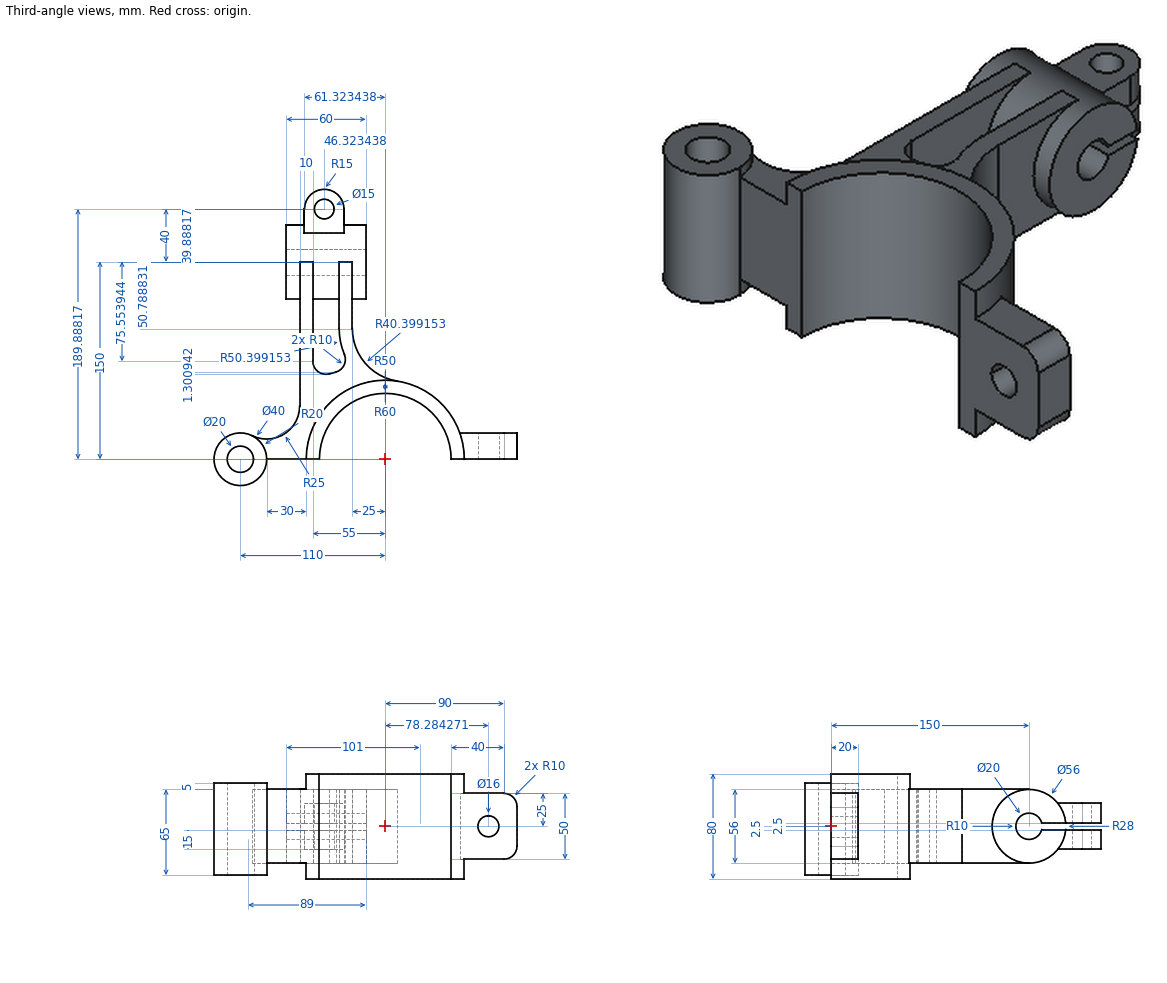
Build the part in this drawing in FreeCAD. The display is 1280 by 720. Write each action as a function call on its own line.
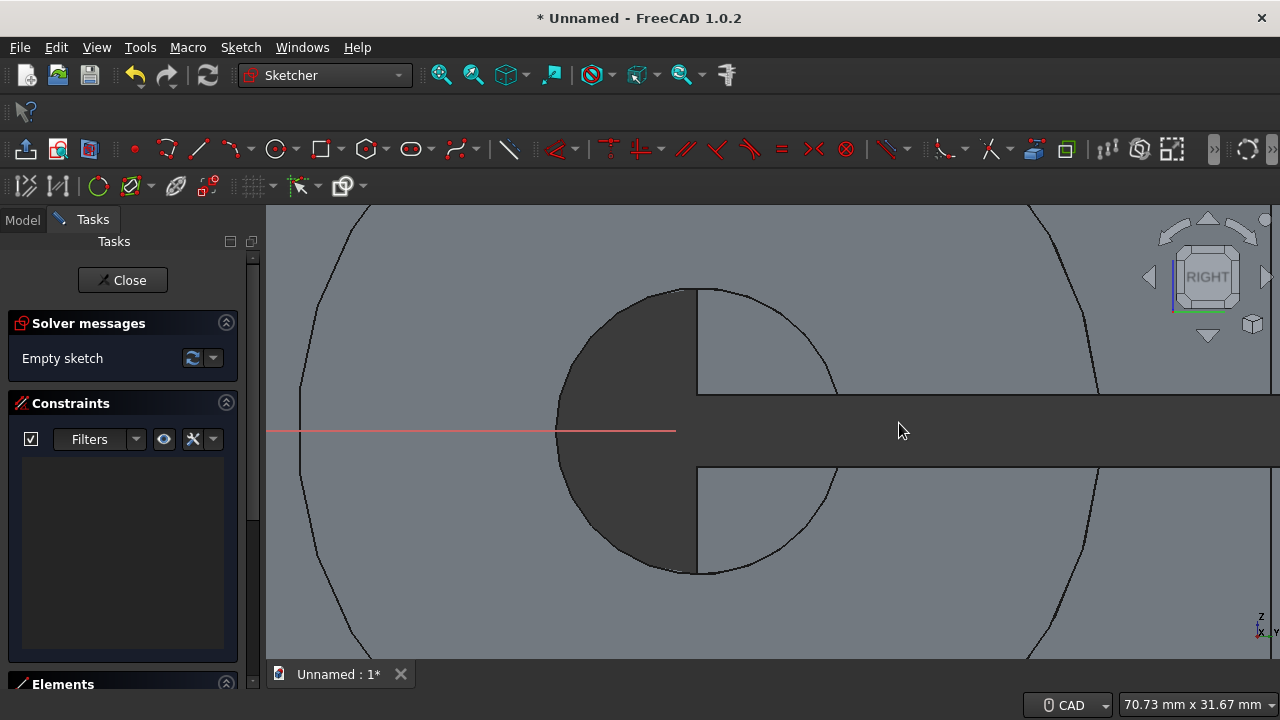
key(g)
key(c)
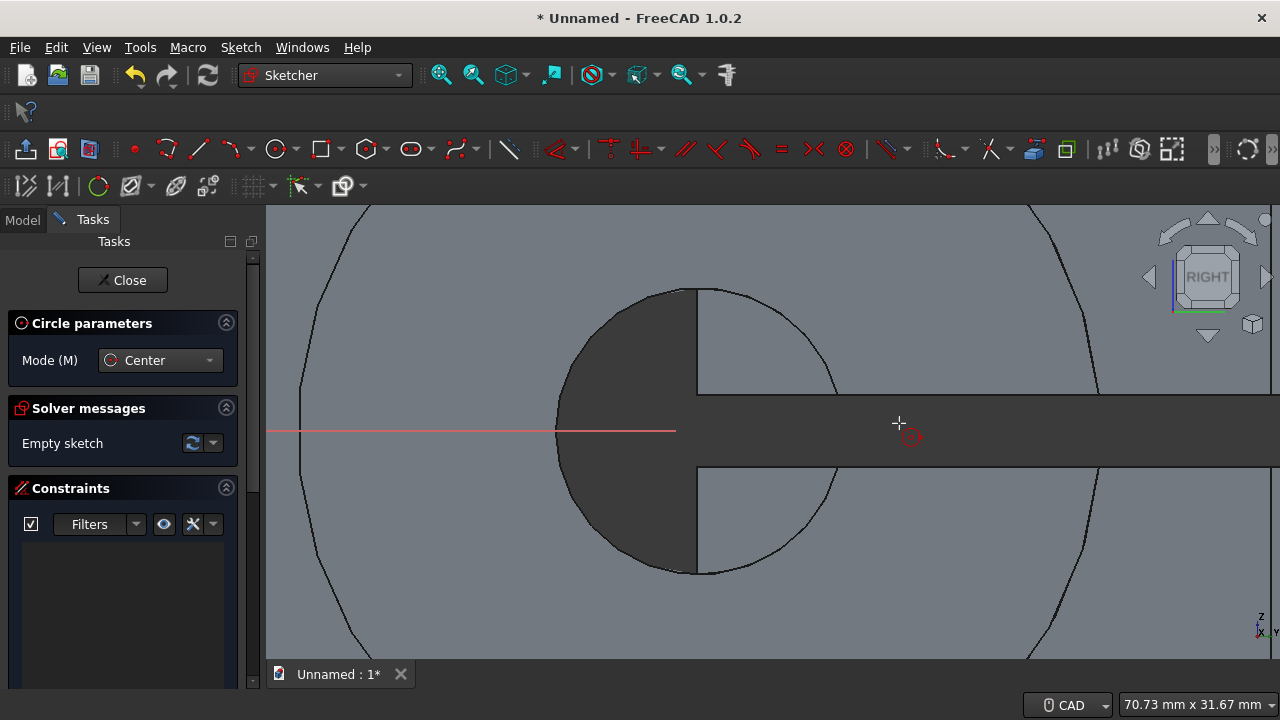
click(699, 431)
move(800, 330)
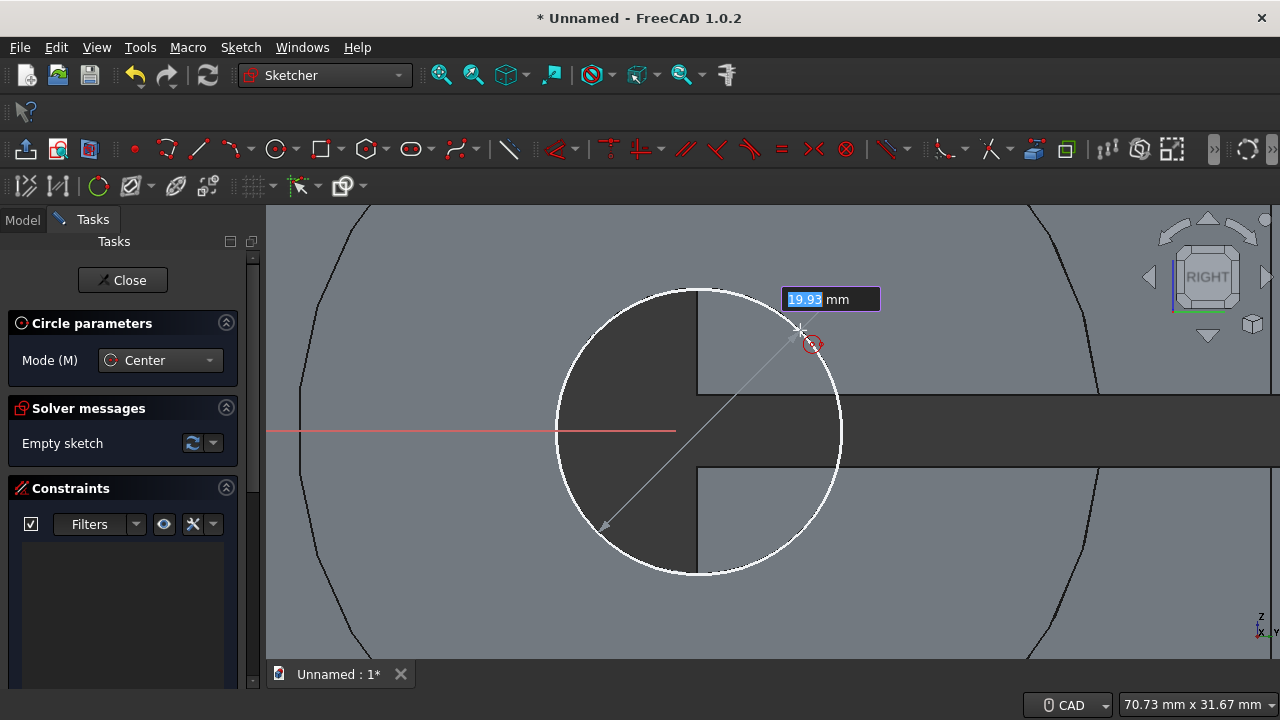
text(20)
key(Return)
key(Escape)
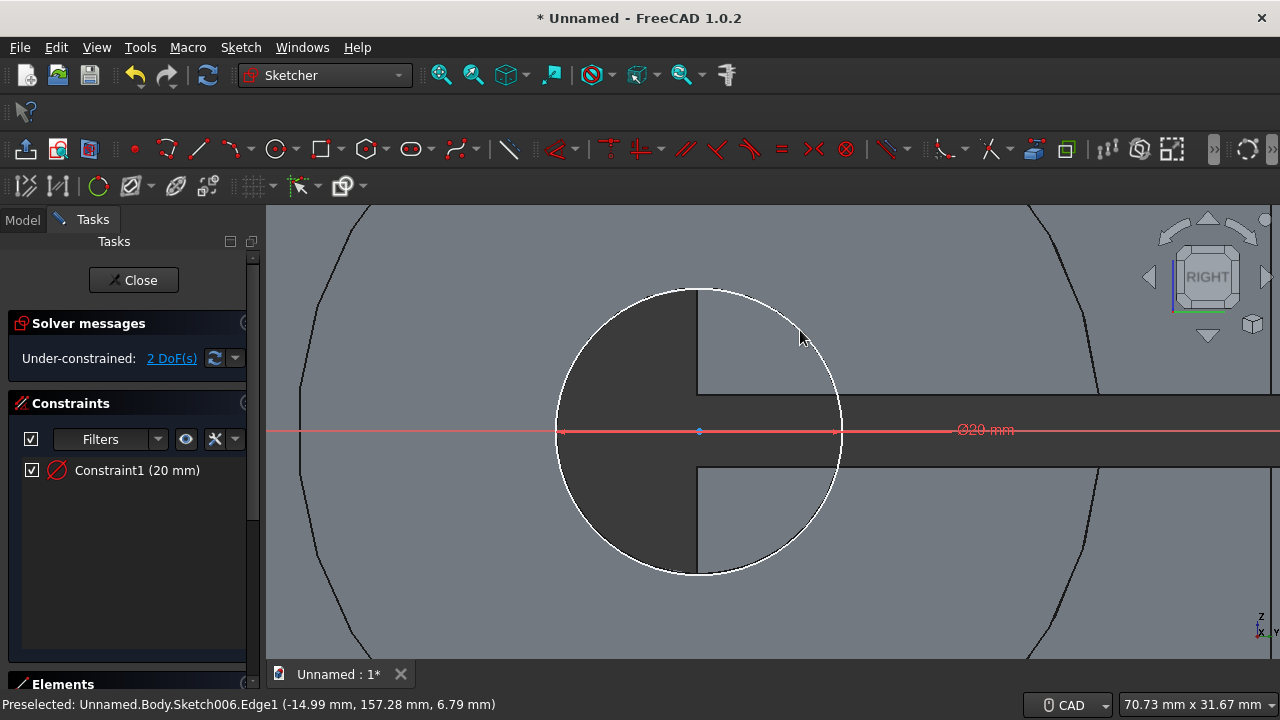
click(699, 432)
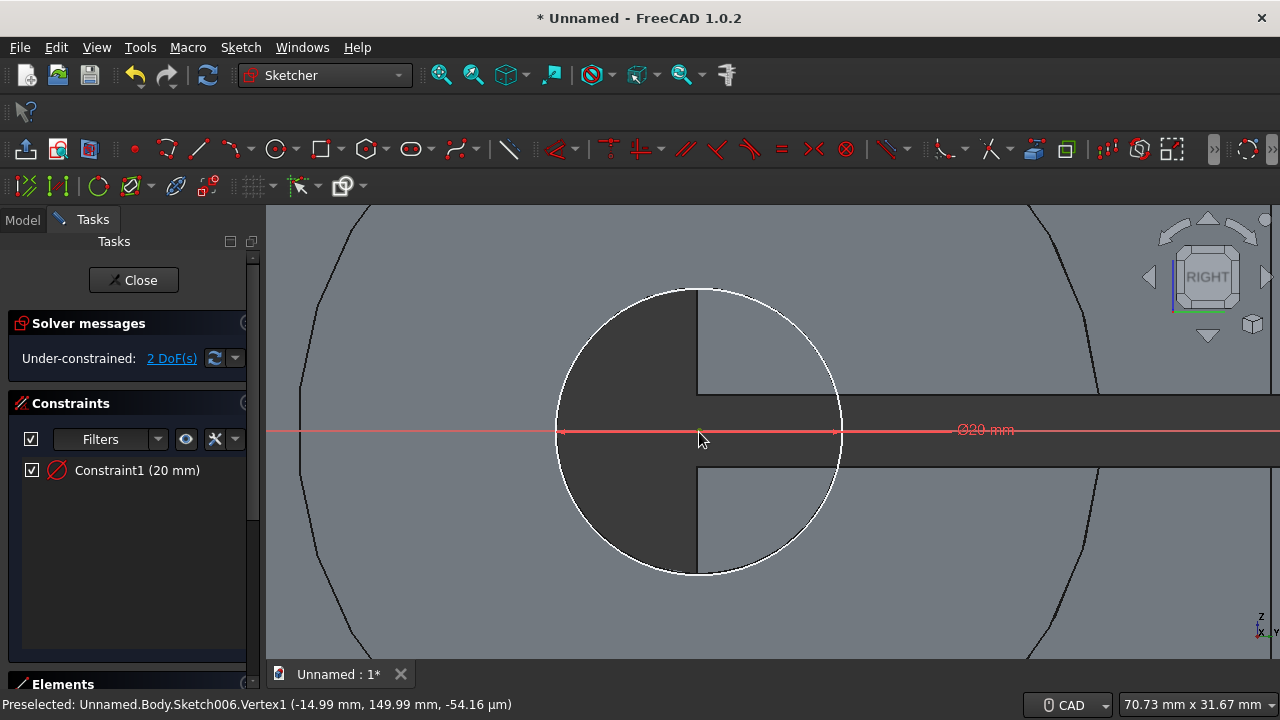
click(353, 431)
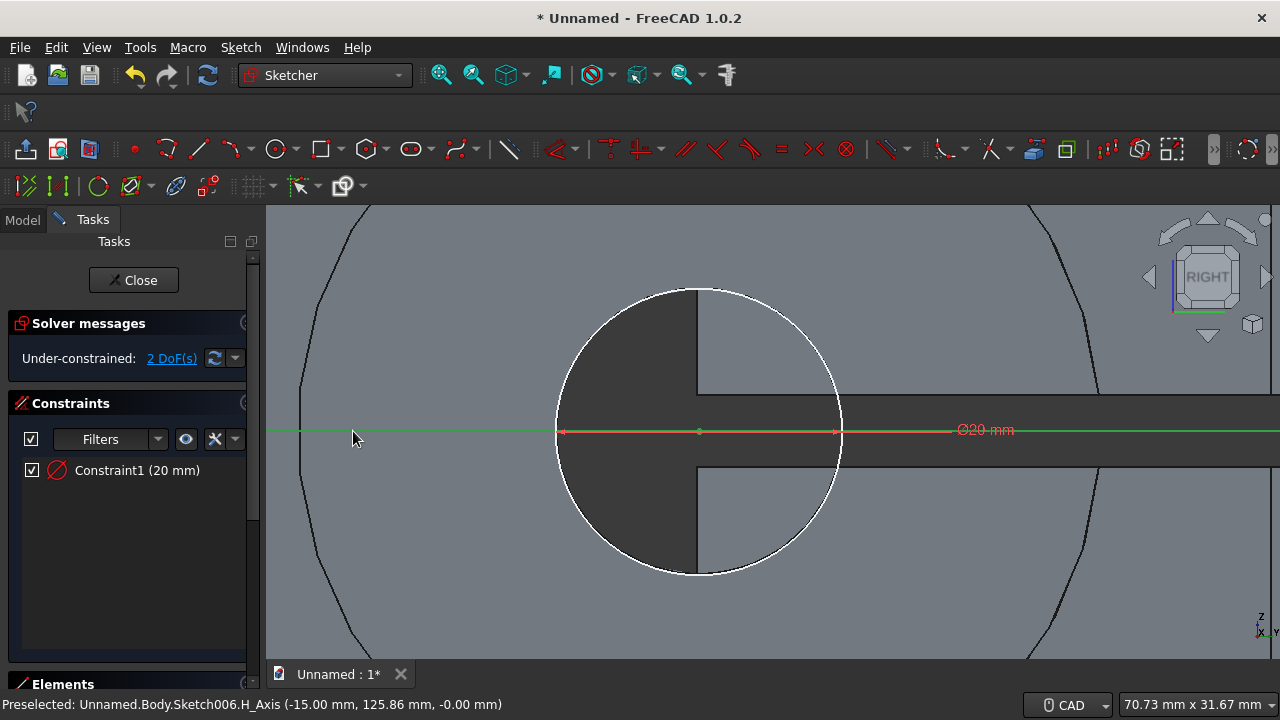
key(c)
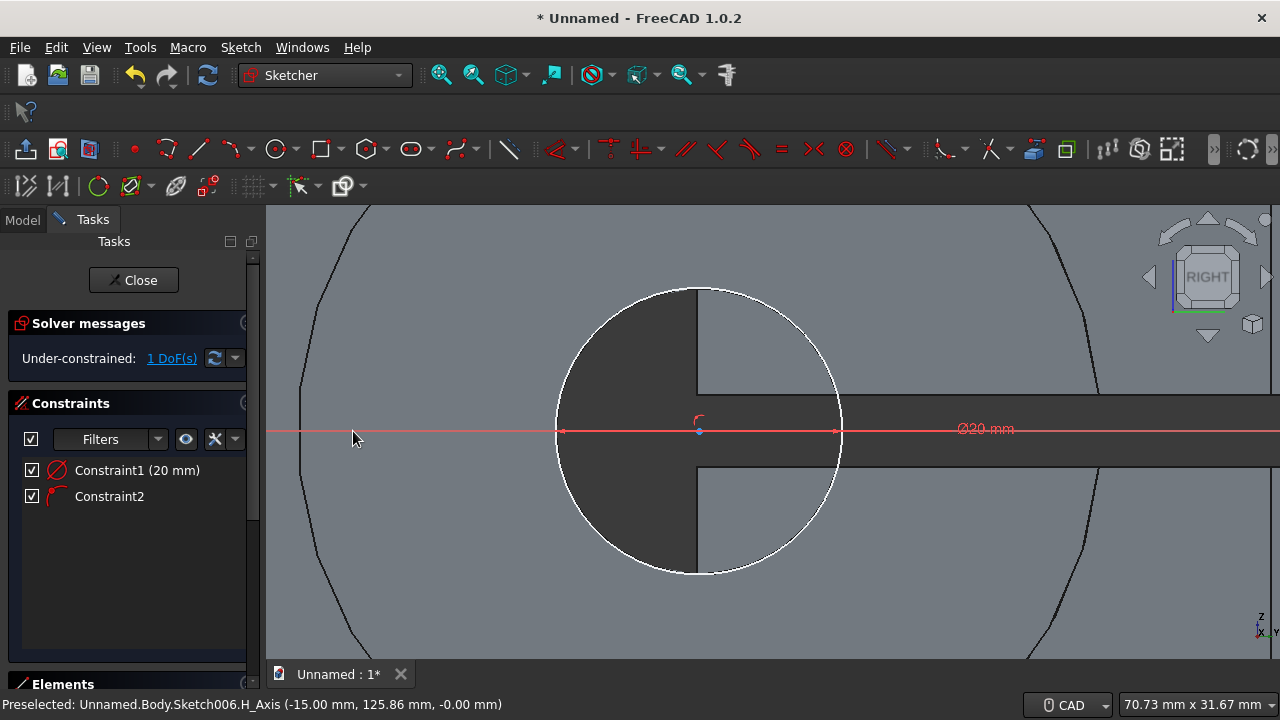
key(d)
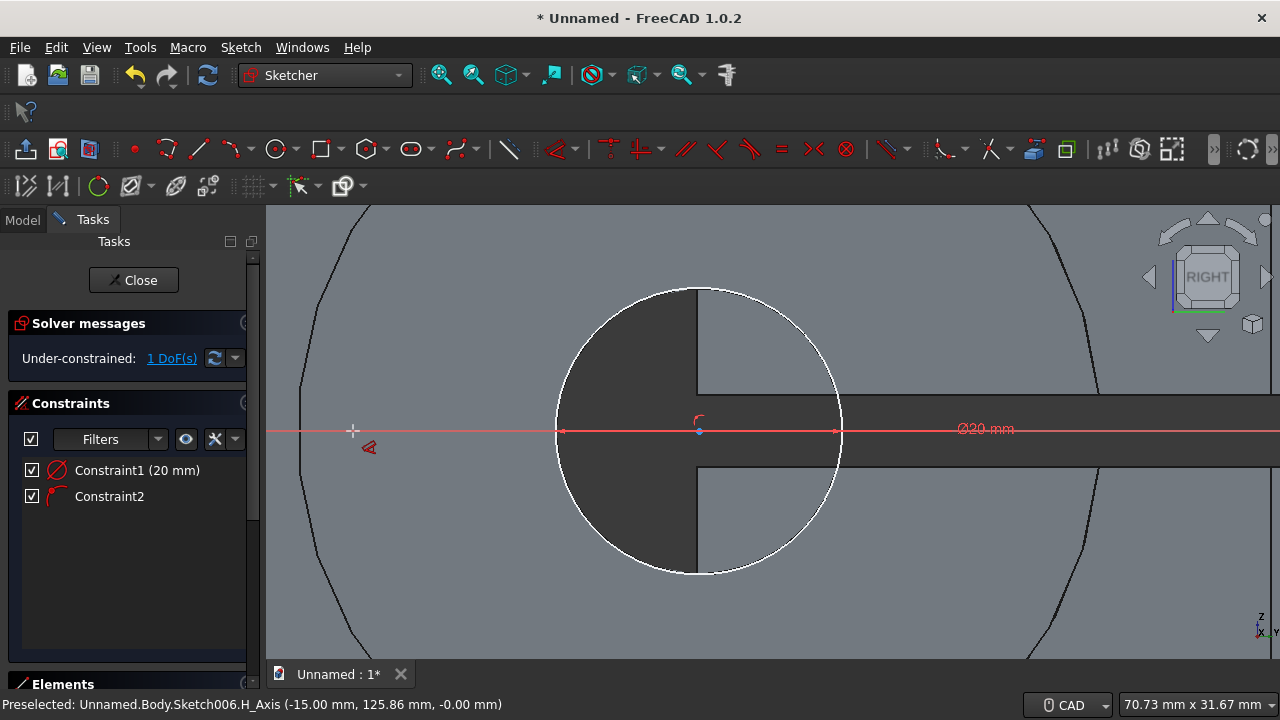
click(699, 431)
click(497, 465)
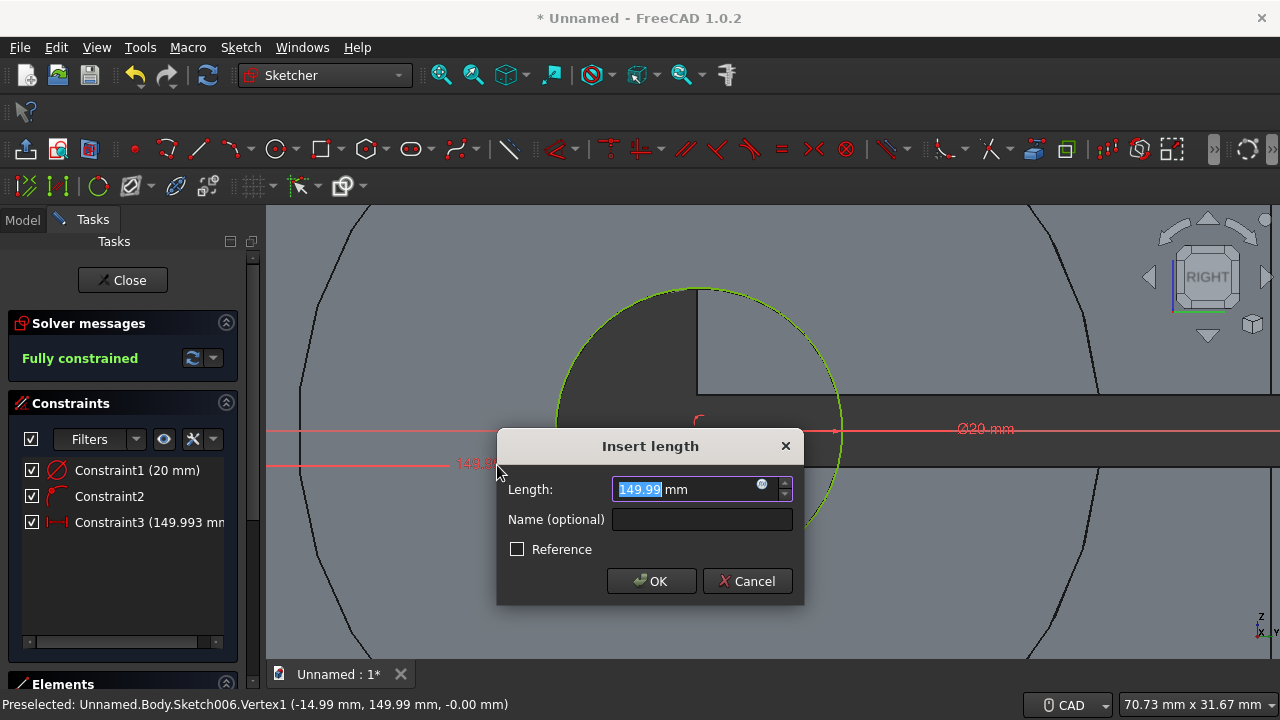
text(150)
key(Return)
key(Escape)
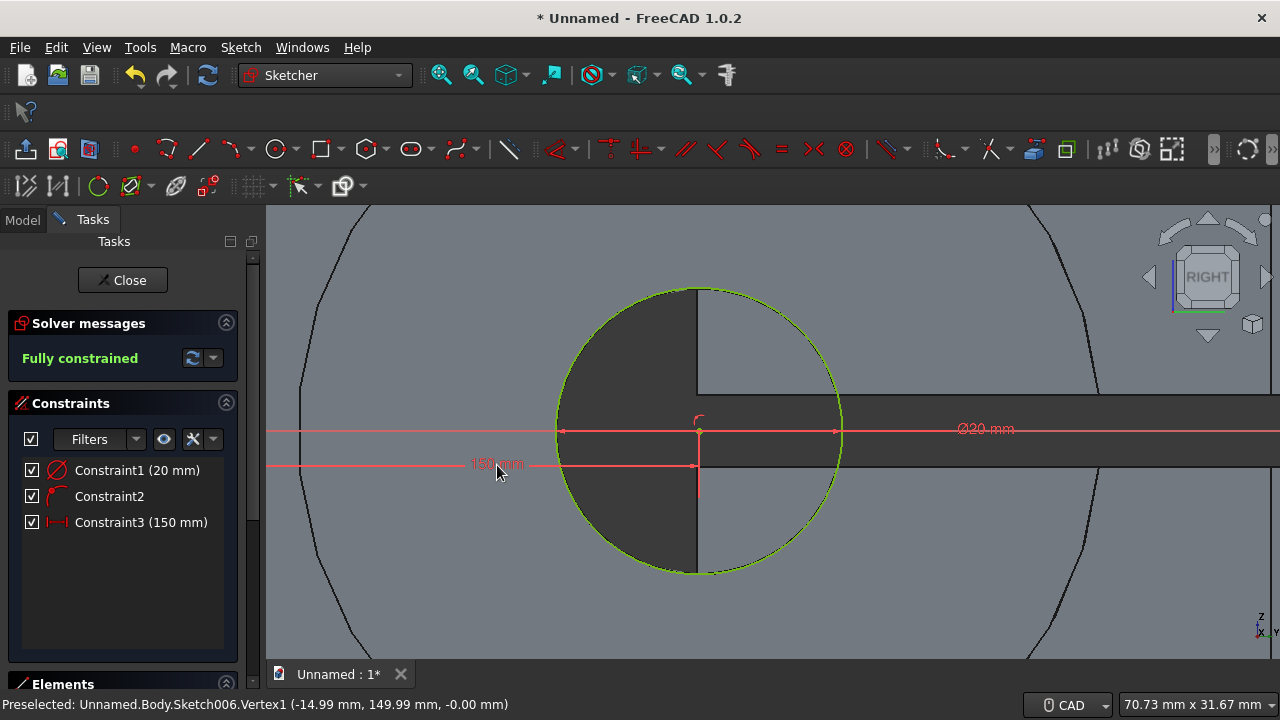
click(123, 280)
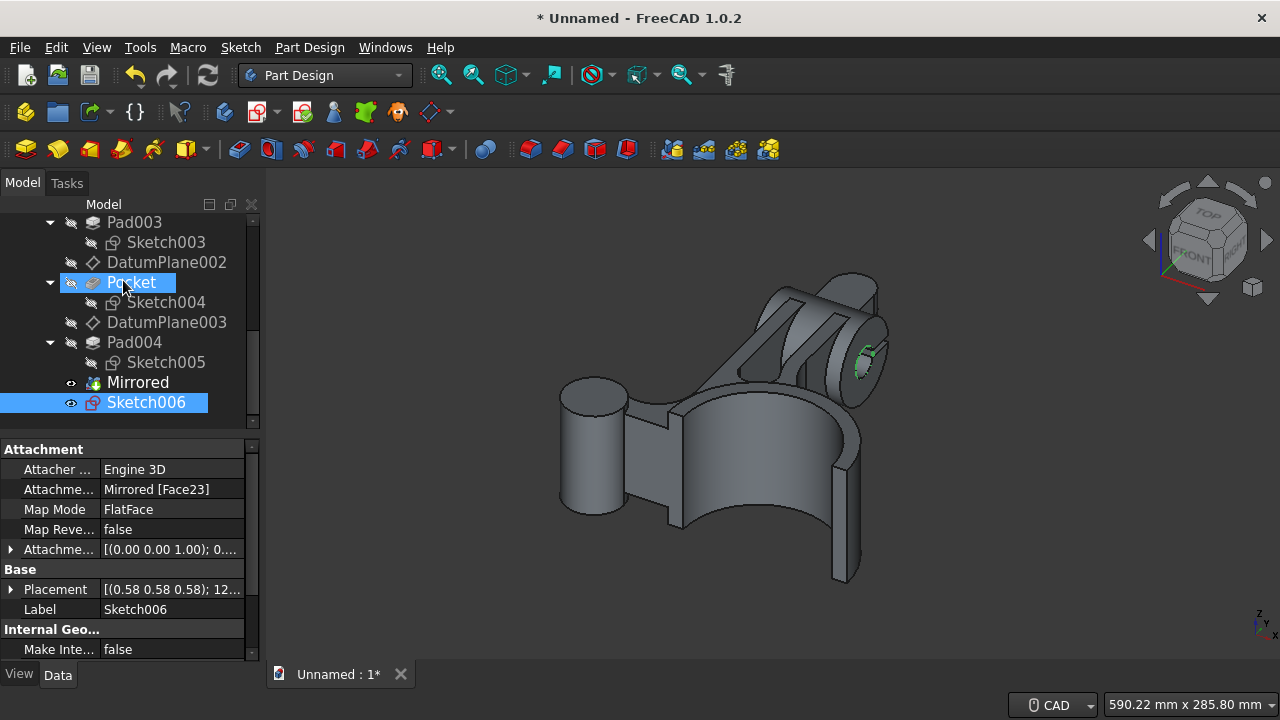
click(240, 150)